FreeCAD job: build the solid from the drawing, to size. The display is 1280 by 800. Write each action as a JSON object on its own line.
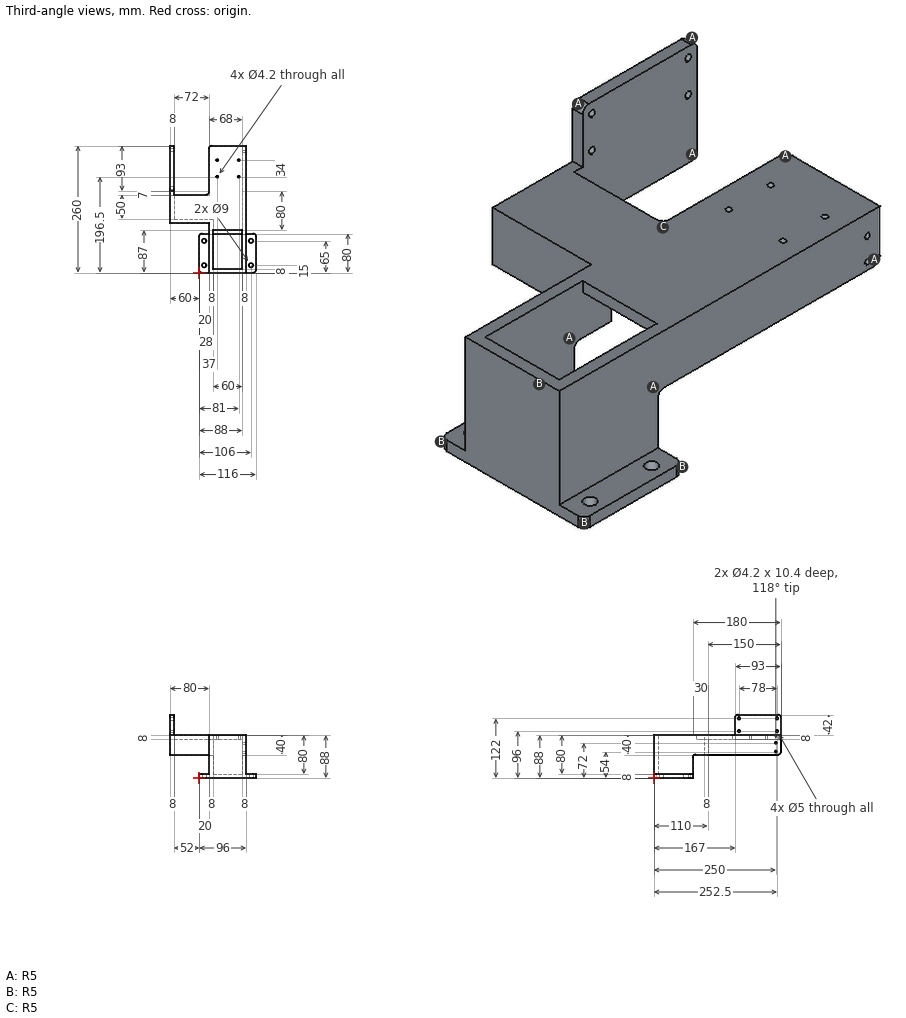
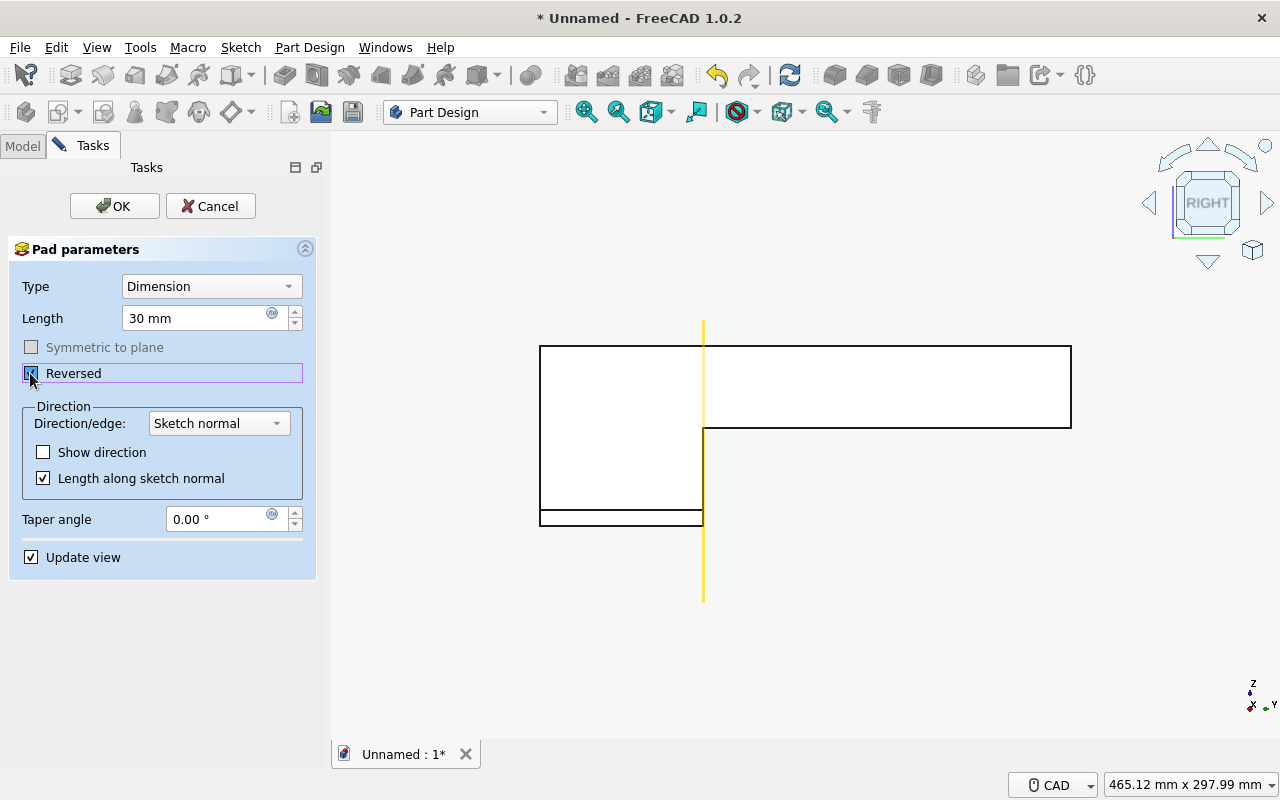
{"action": "left_click", "coordinate": [115, 206]}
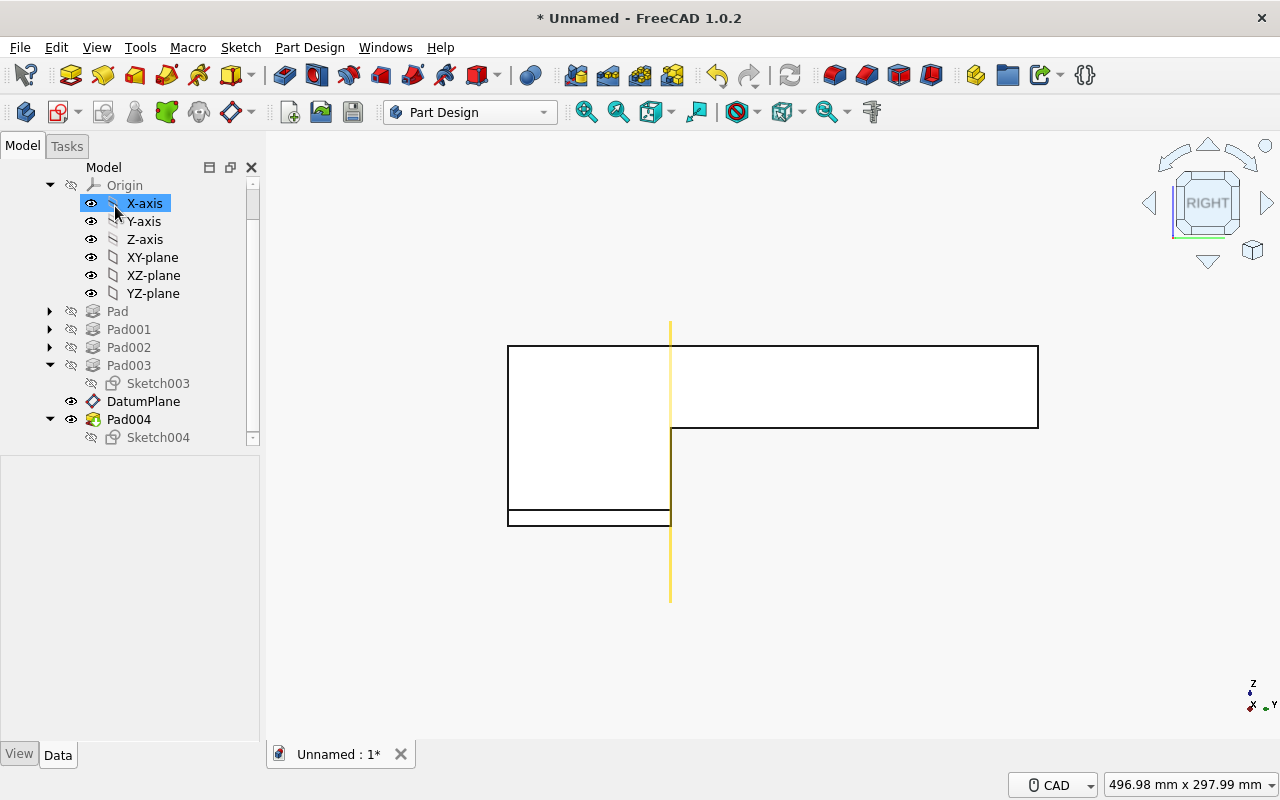
{"action": "left_click", "coordinate": [116, 401]}
{"action": "key", "text": "space"}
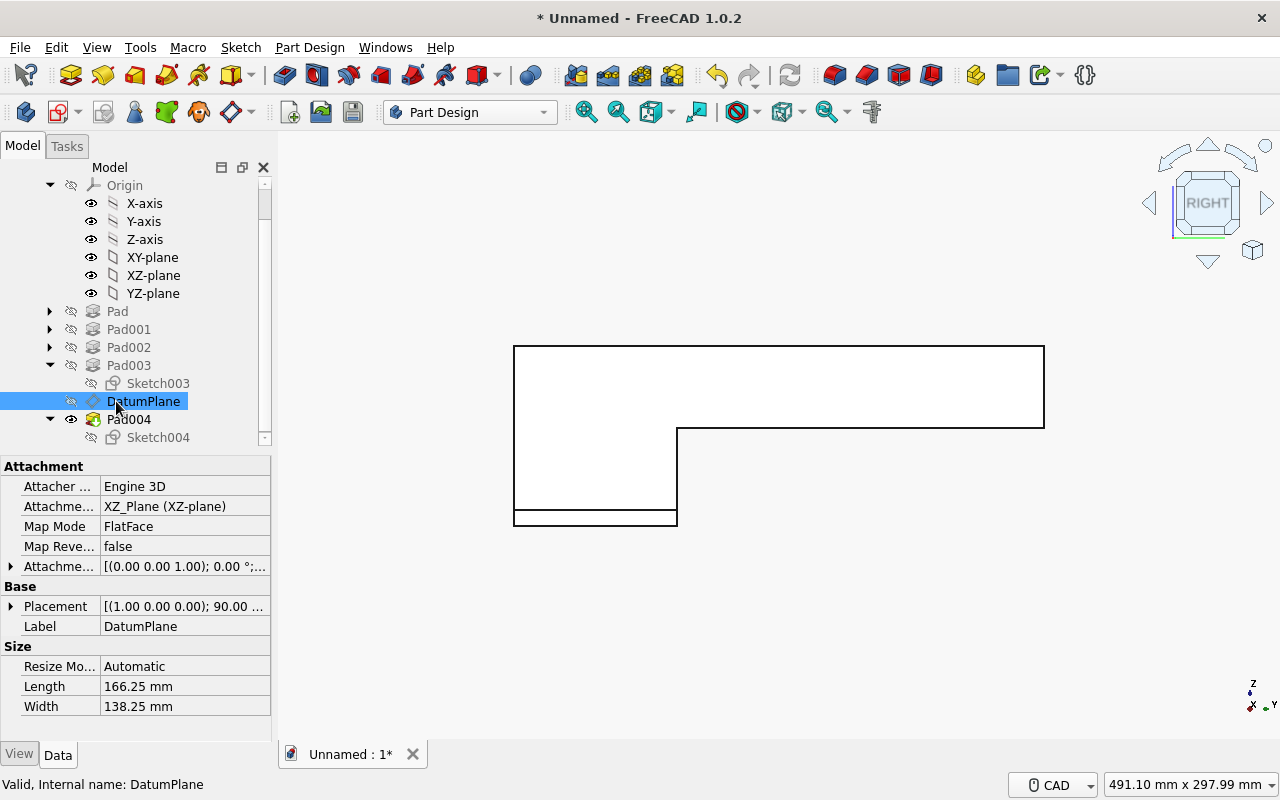
{"action": "key", "text": "6"}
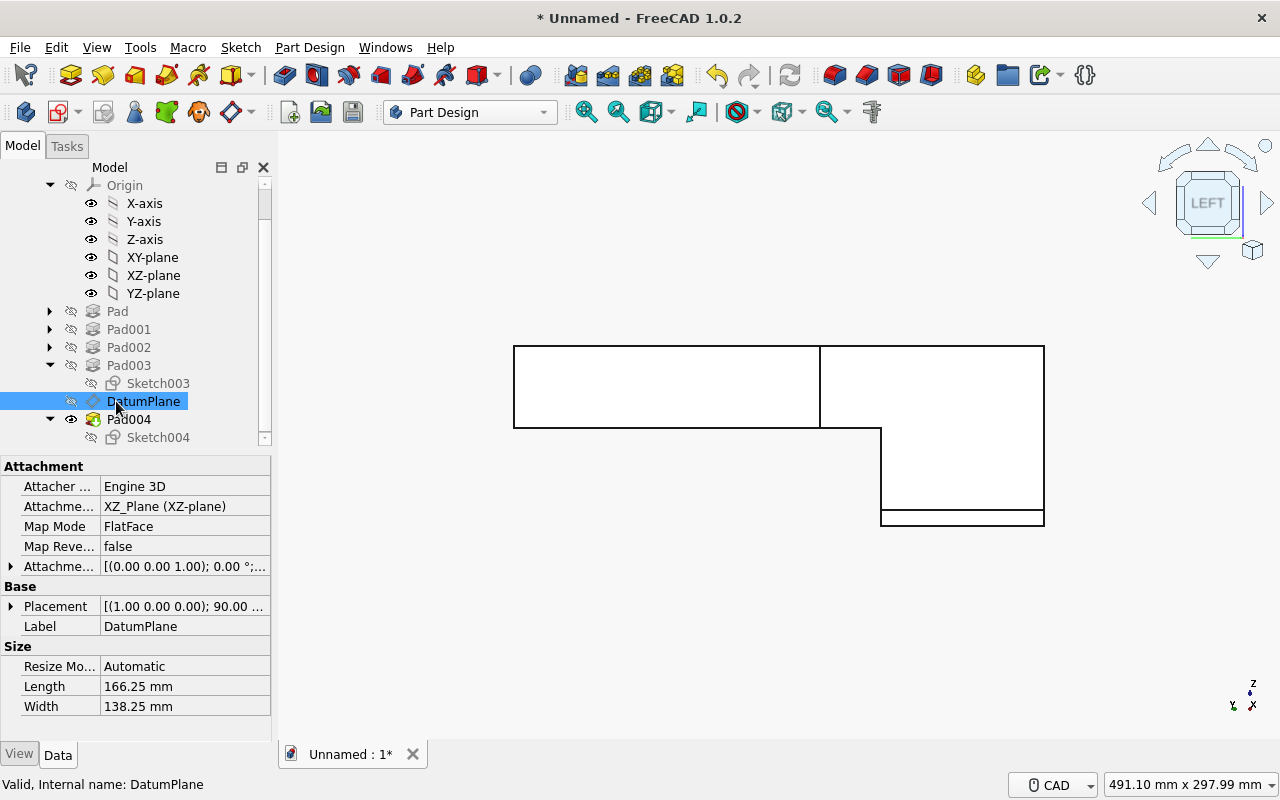
{"action": "left_click", "coordinate": [964, 427]}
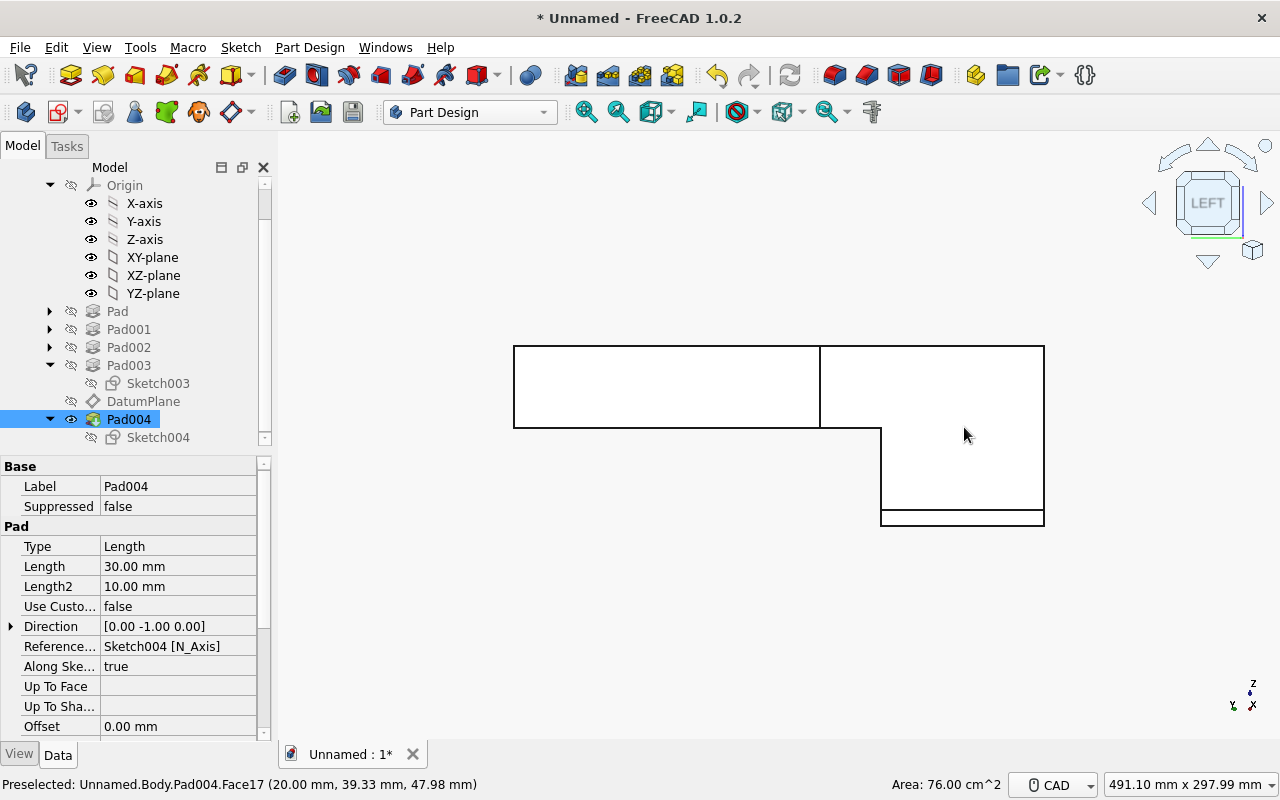
{"action": "left_click", "coordinate": [58, 112]}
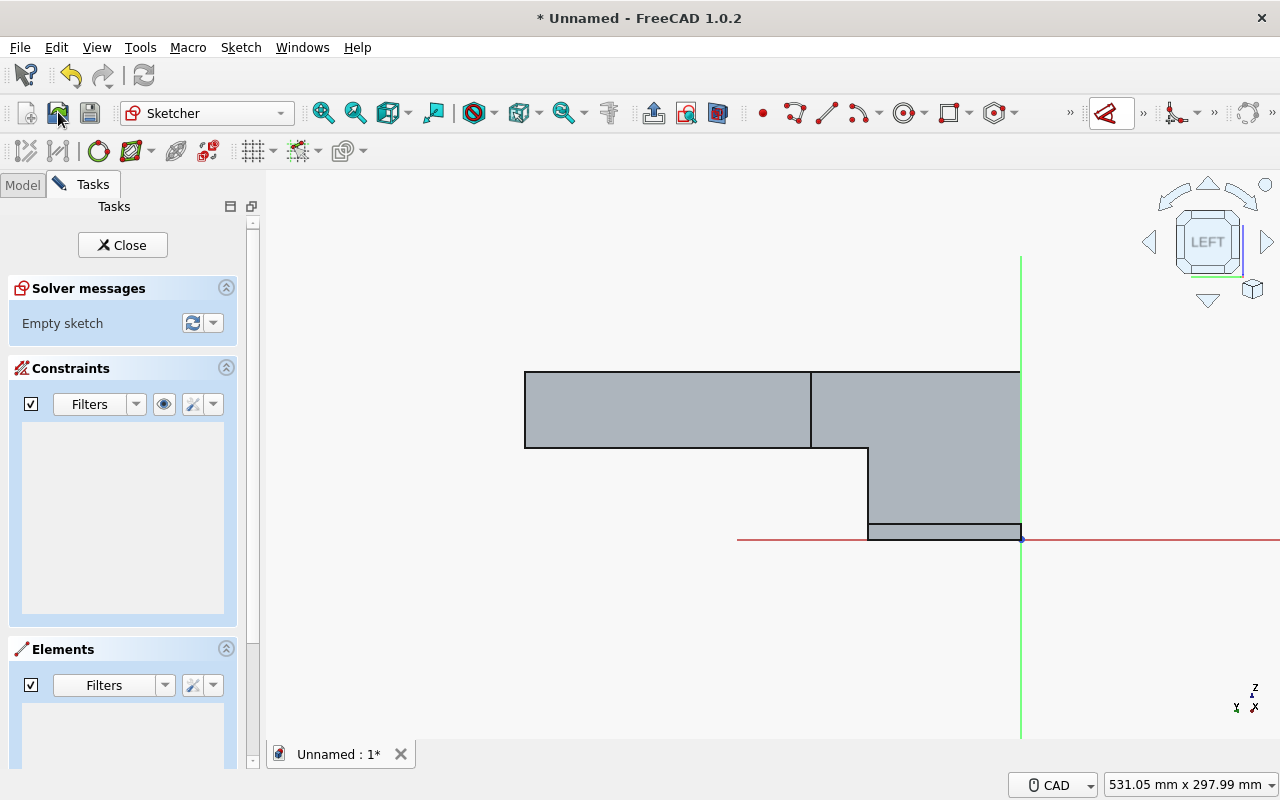
{"action": "left_click", "coordinate": [718, 114]}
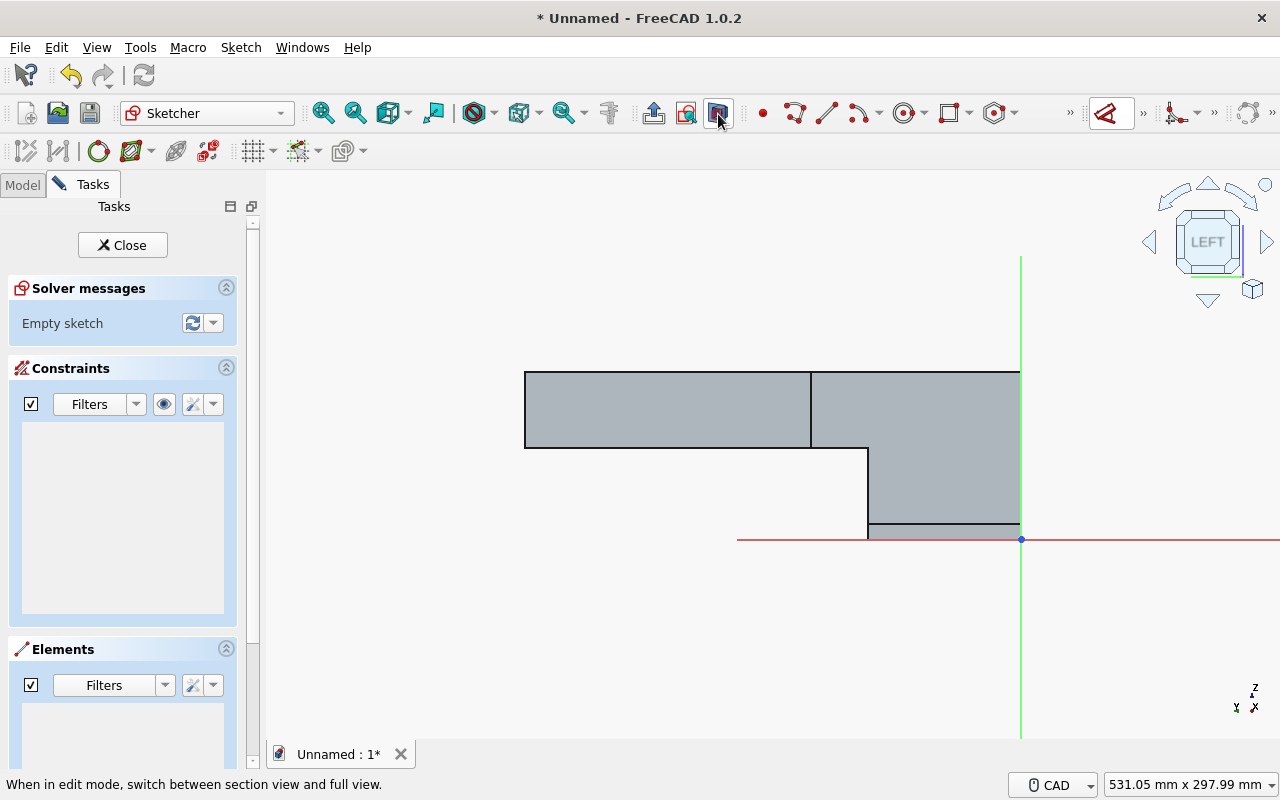
{"action": "scroll", "coordinate": [848, 398], "scroll_direction": "up", "scroll_amount": 8}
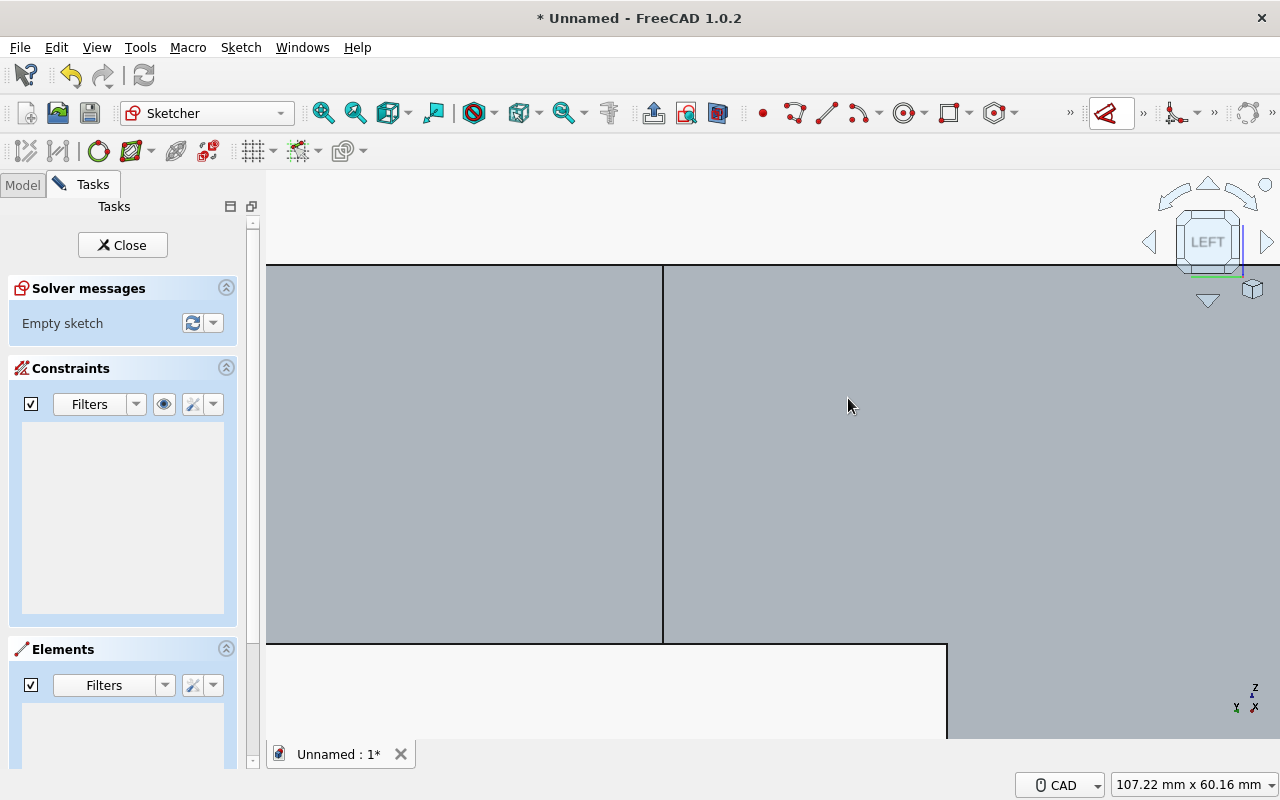
{"action": "left_click", "coordinate": [950, 114]}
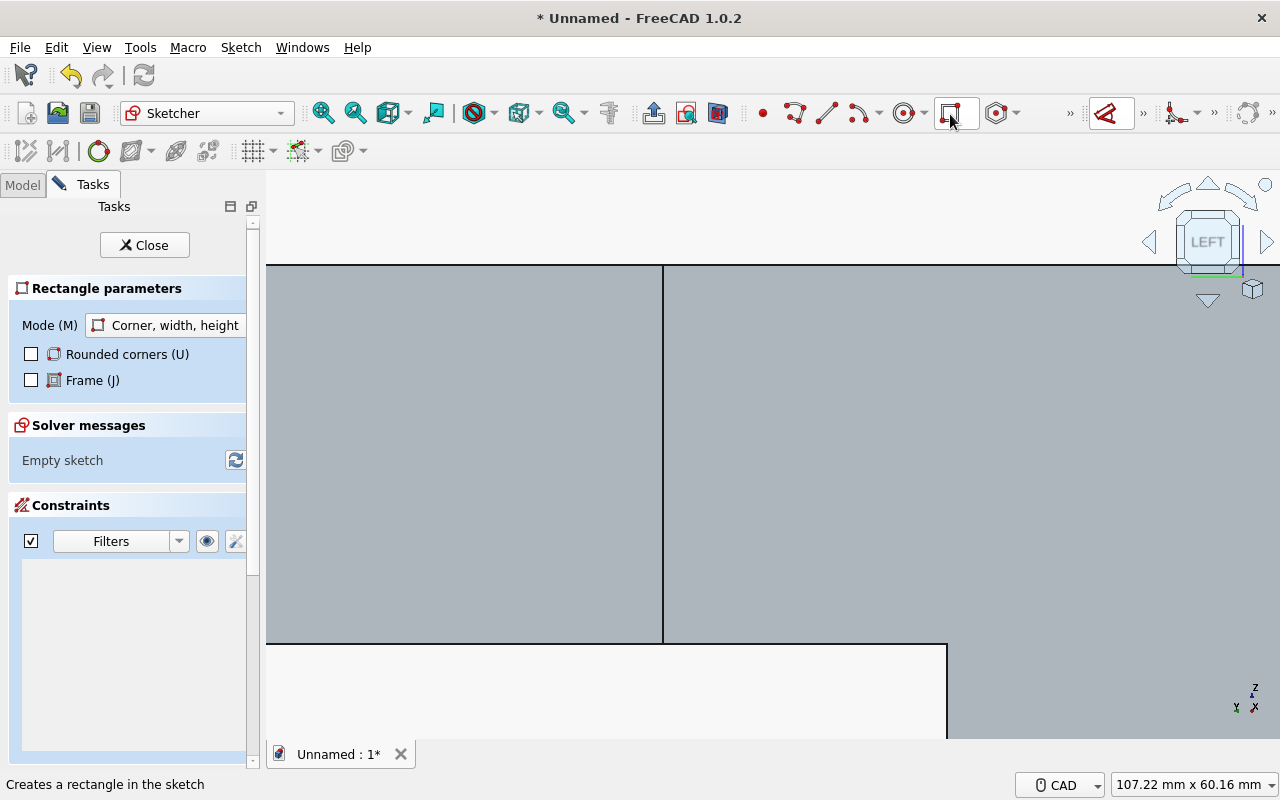
{"action": "left_click", "coordinate": [663, 265]}
{"action": "left_click", "coordinate": [739, 644]}
{"action": "key", "text": "Escape"}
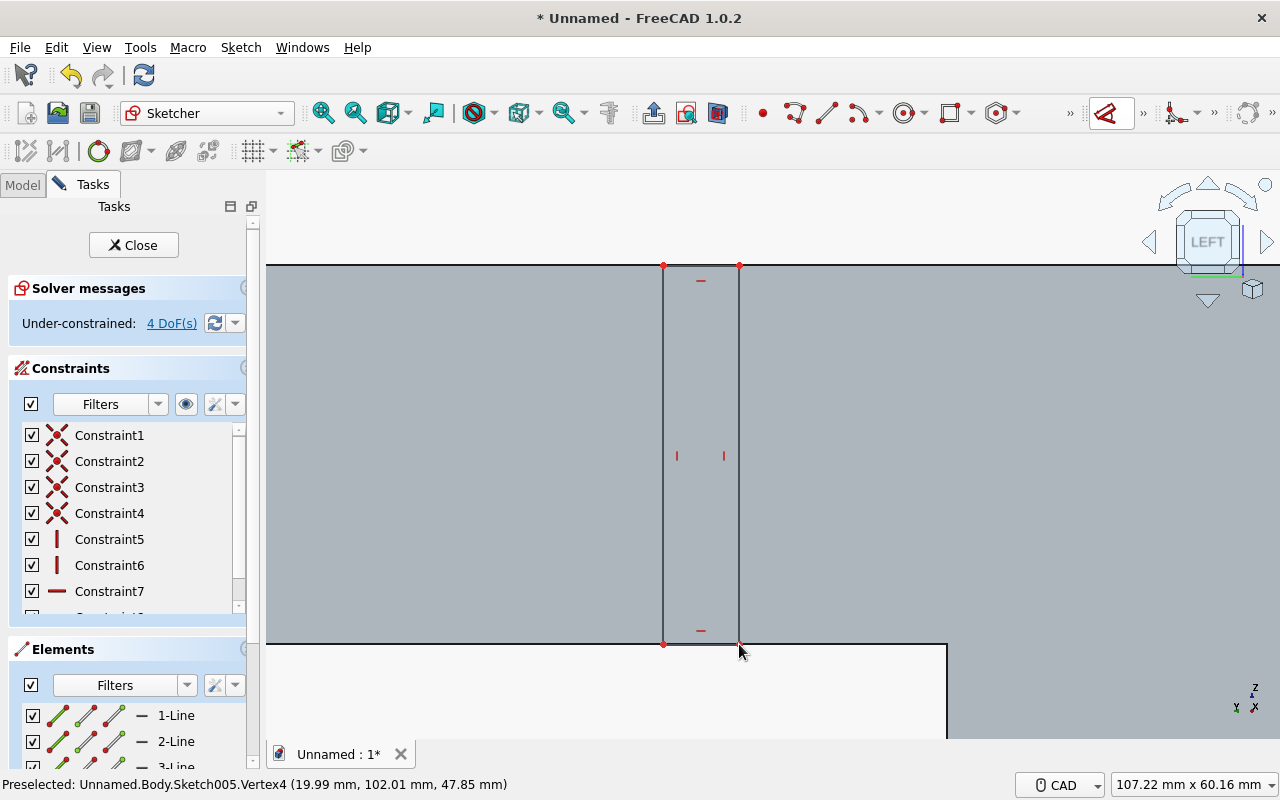
{"action": "left_click", "coordinate": [686, 645]}